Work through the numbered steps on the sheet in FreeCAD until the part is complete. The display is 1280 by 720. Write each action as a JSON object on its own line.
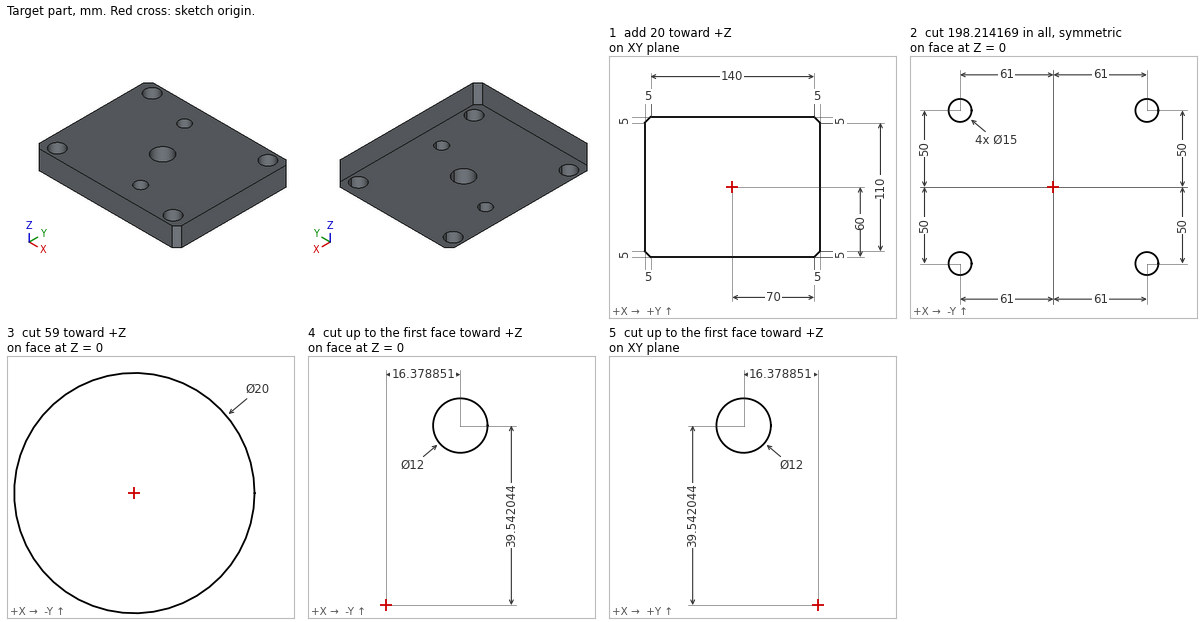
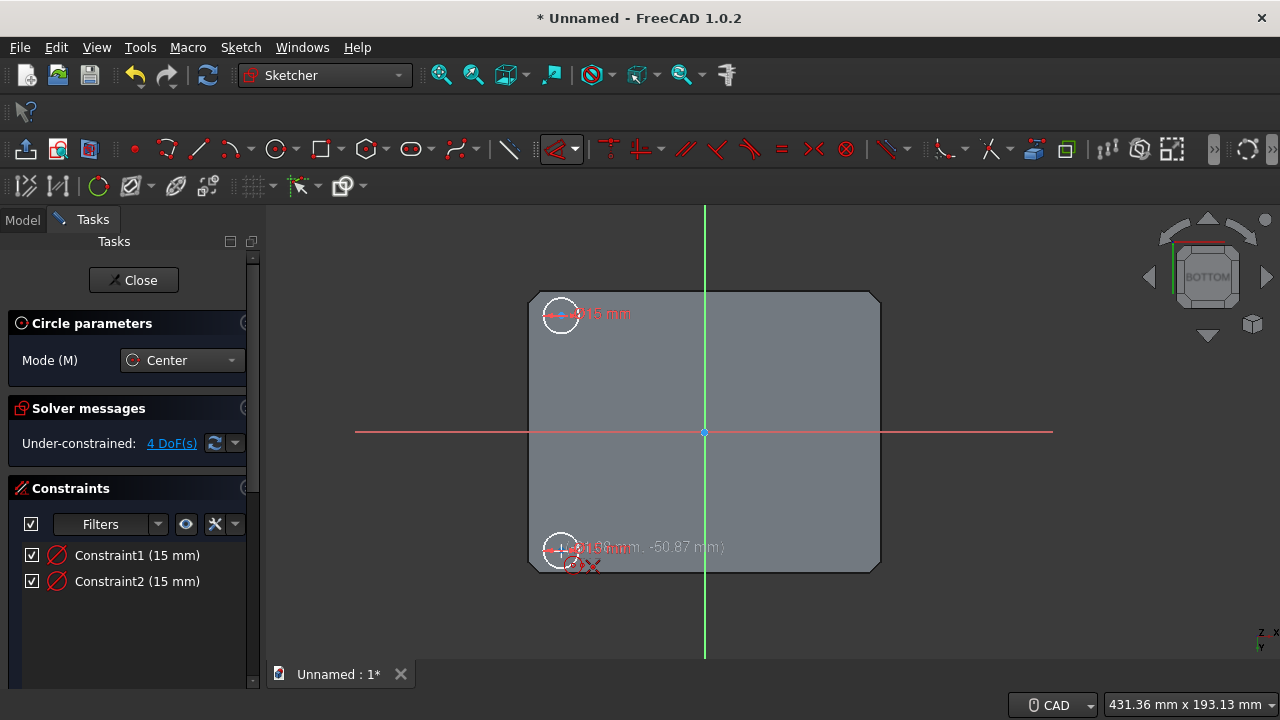
{"action": "scroll", "coordinate": [848, 315], "scroll_direction": "up", "scroll_amount": 2}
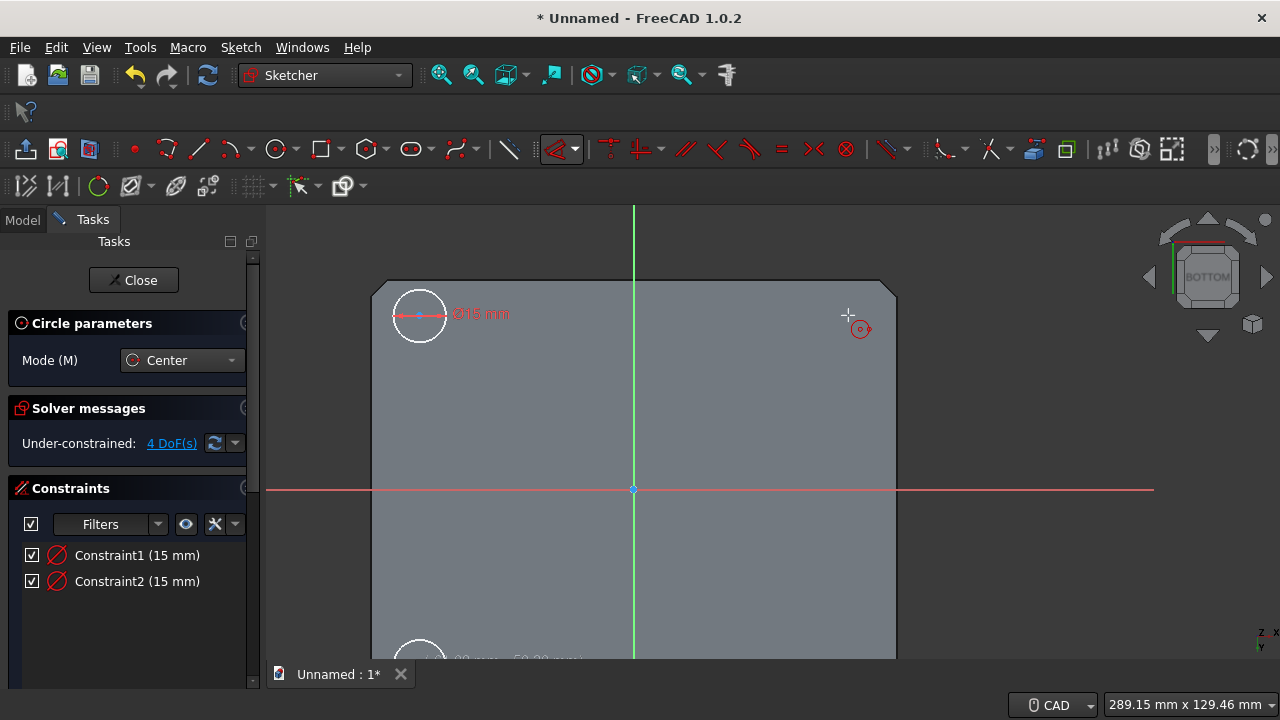
{"action": "left_click", "coordinate": [848, 315]}
{"action": "mouse_move", "coordinate": [866, 296]}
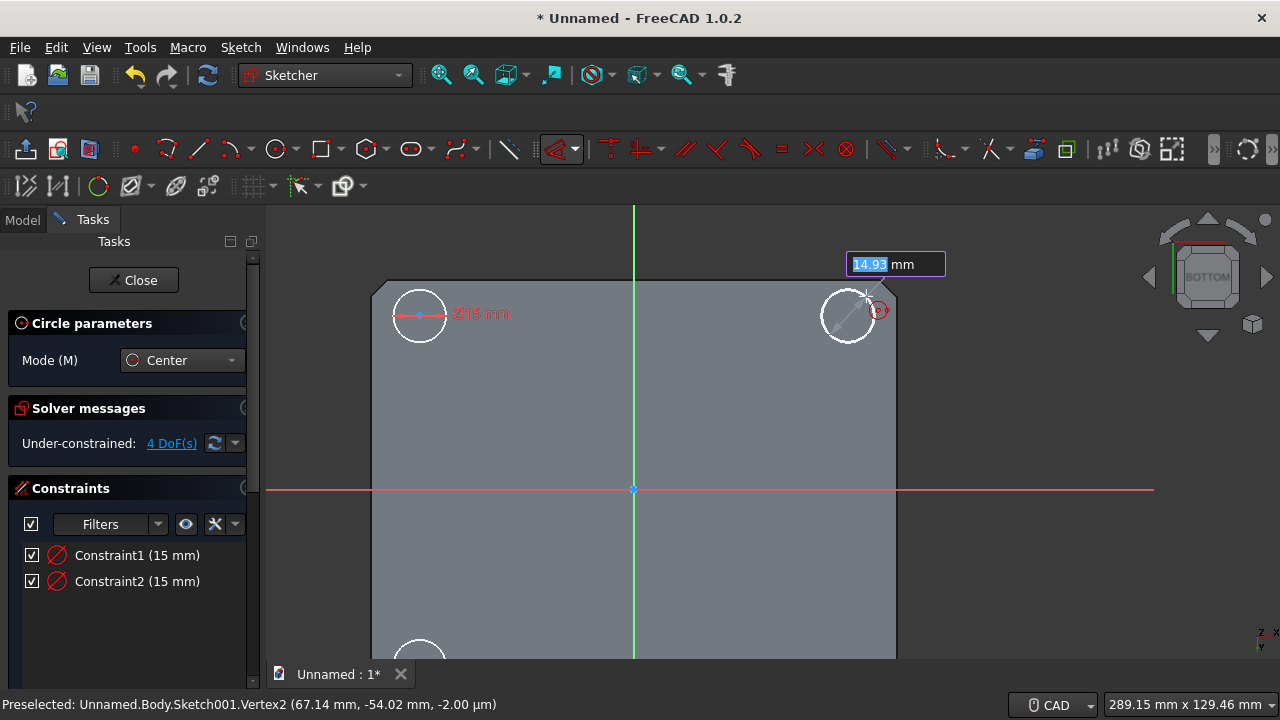
{"action": "type", "text": "15"}
{"action": "key", "text": "Return"}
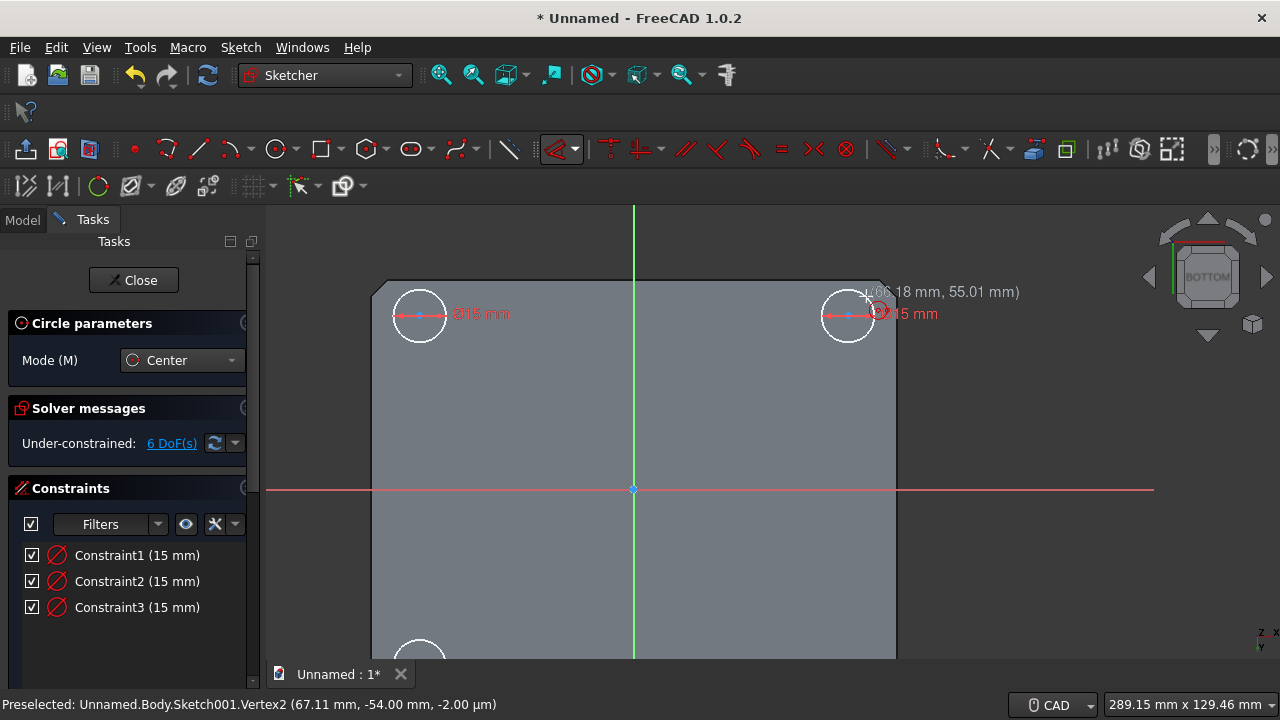
{"action": "scroll", "coordinate": [848, 314], "scroll_direction": "down", "scroll_amount": 2}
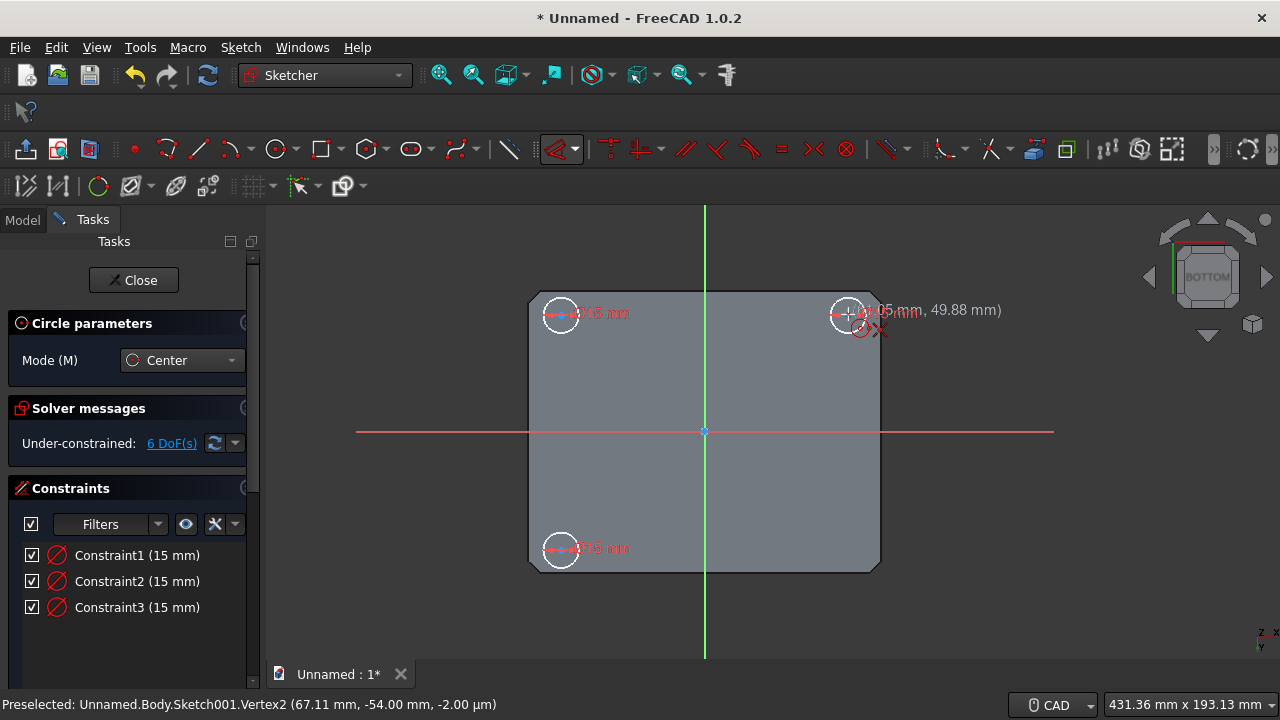
{"action": "scroll", "coordinate": [848, 550], "scroll_direction": "up", "scroll_amount": 2}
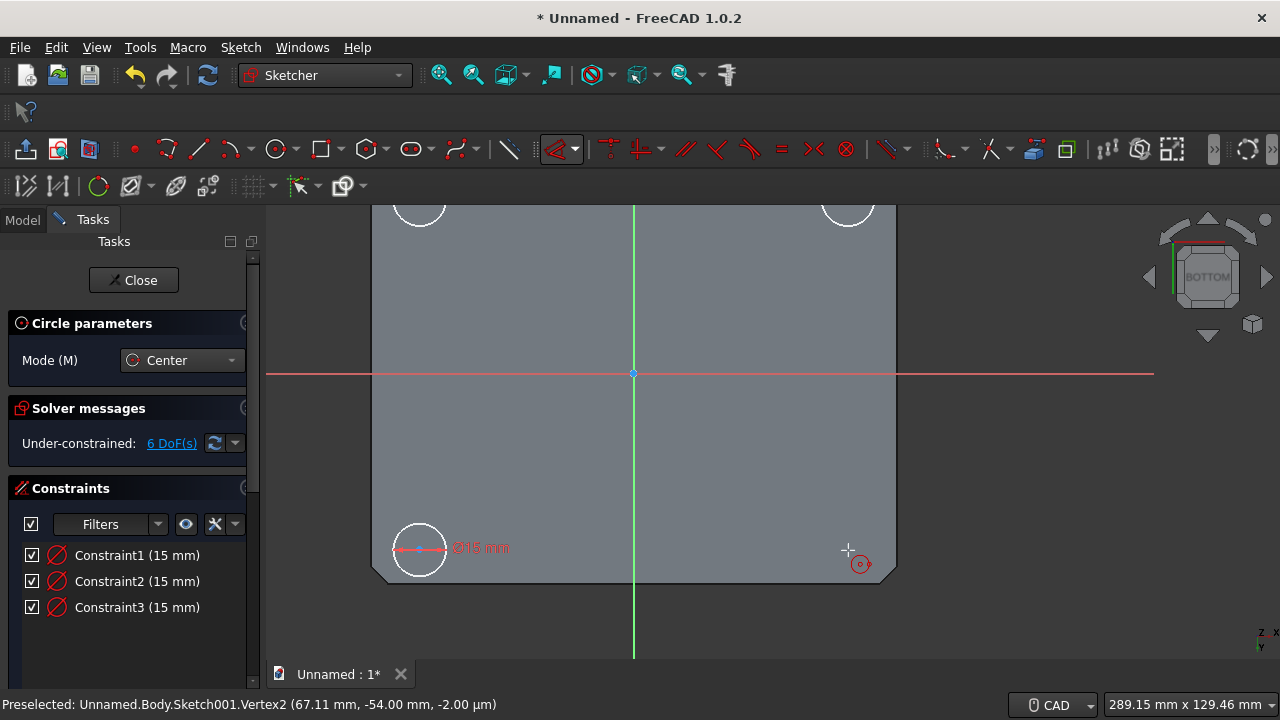
{"action": "left_click", "coordinate": [848, 549]}
{"action": "mouse_move", "coordinate": [866, 530]}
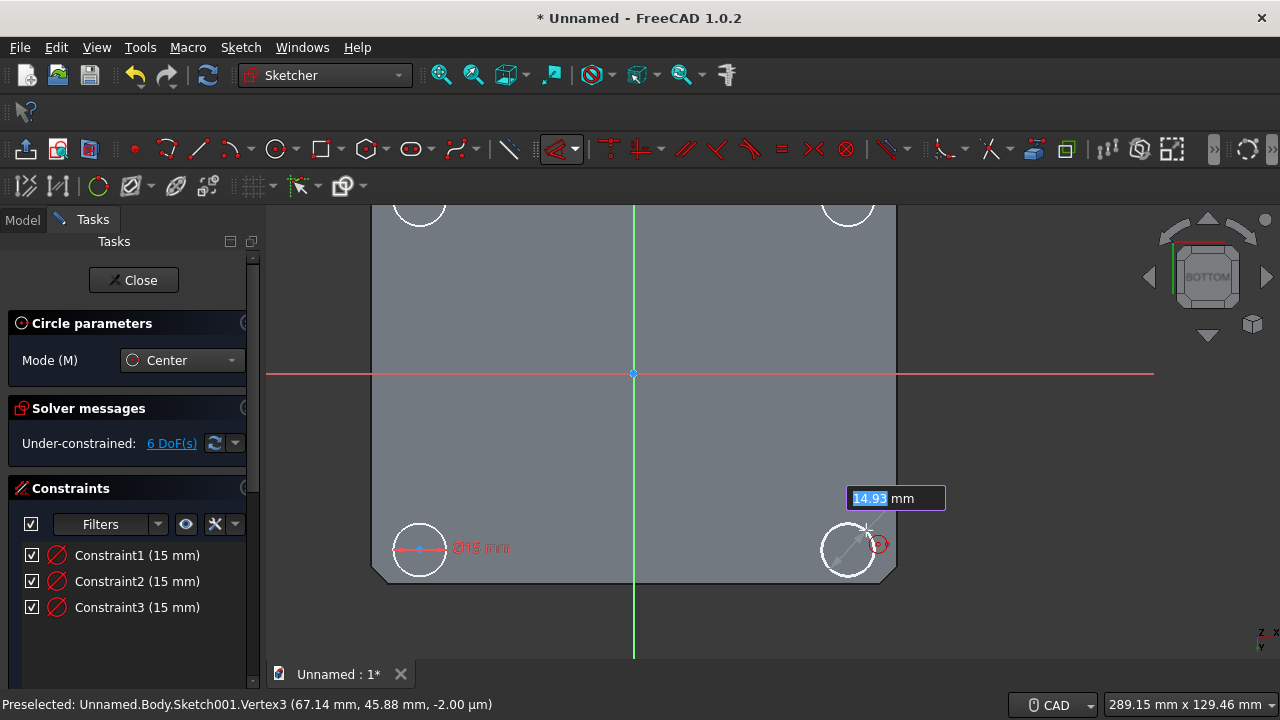
{"action": "type", "text": "15"}
{"action": "key", "text": "Return"}
{"action": "key", "text": "Escape"}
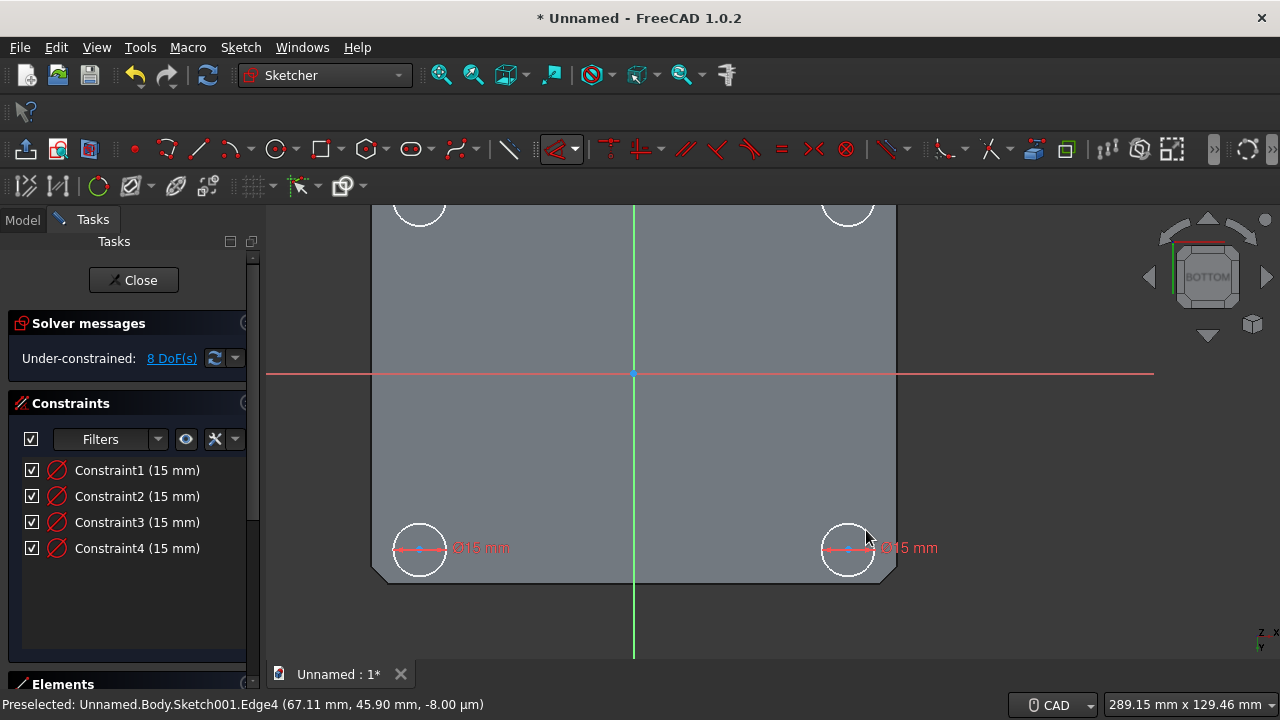
{"action": "scroll", "coordinate": [848, 551], "scroll_direction": "down", "scroll_amount": 2}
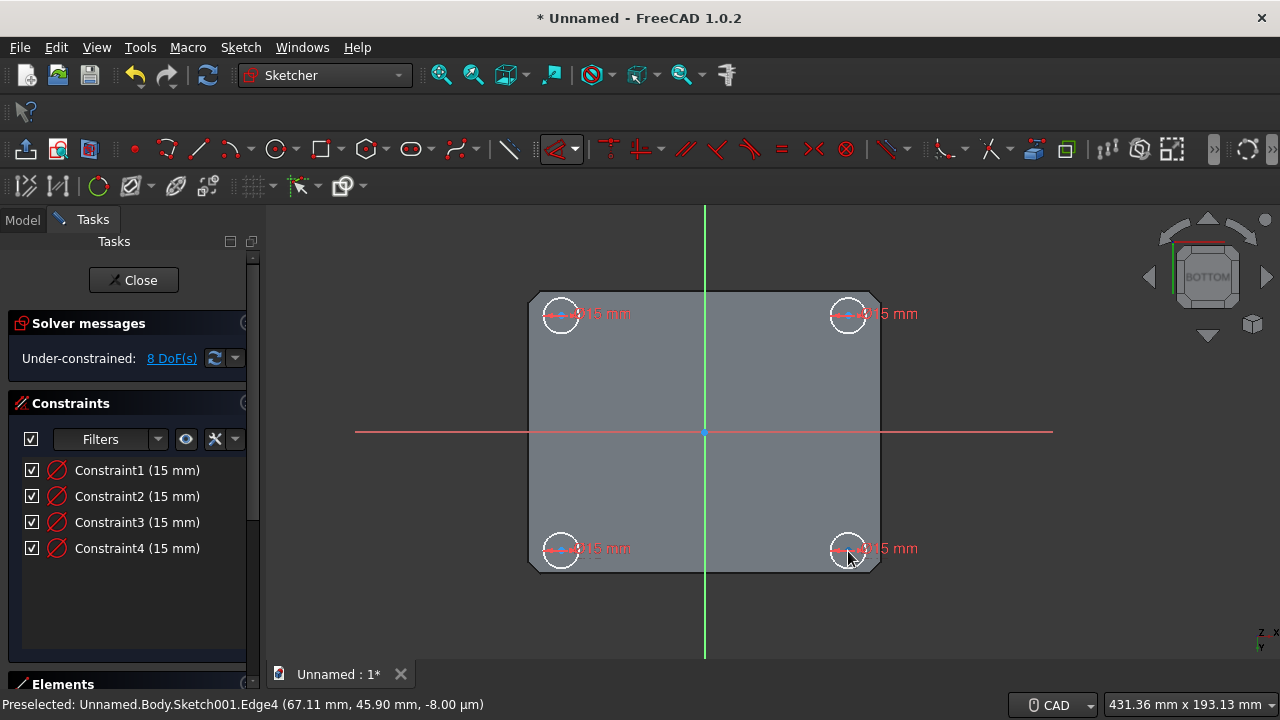
{"action": "left_click", "coordinate": [561, 316]}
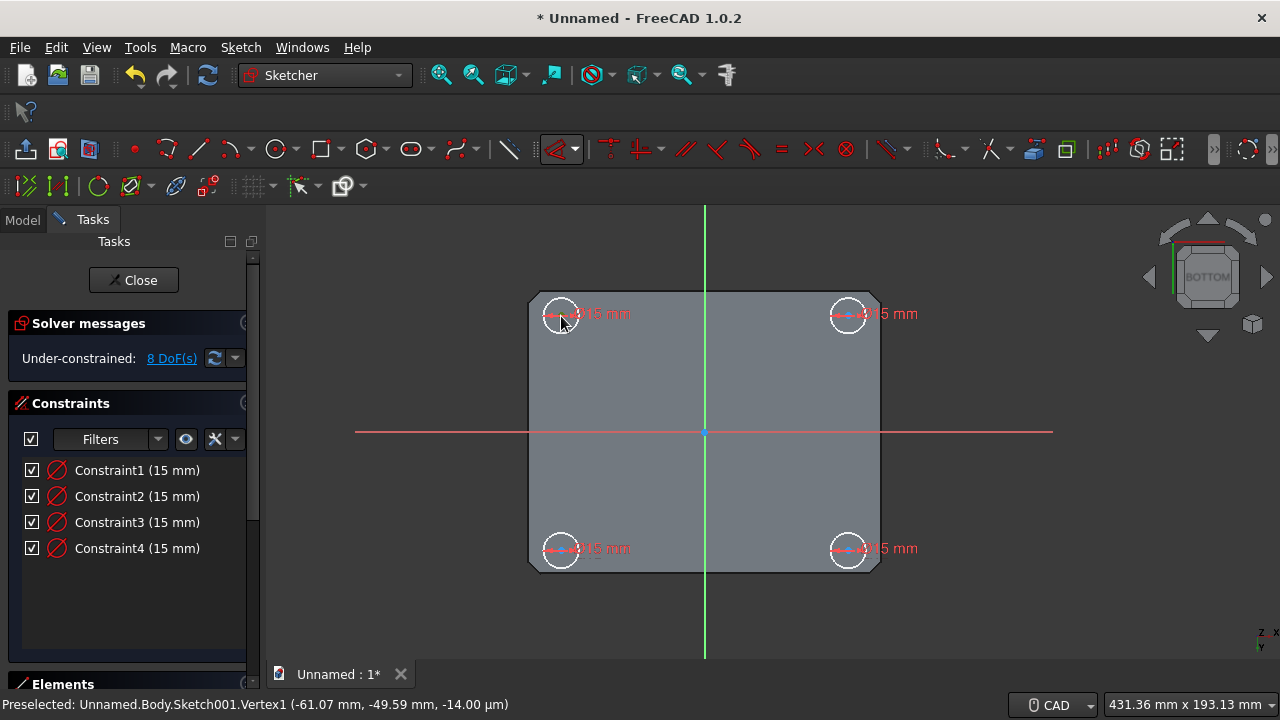
{"action": "left_click", "coordinate": [578, 150]}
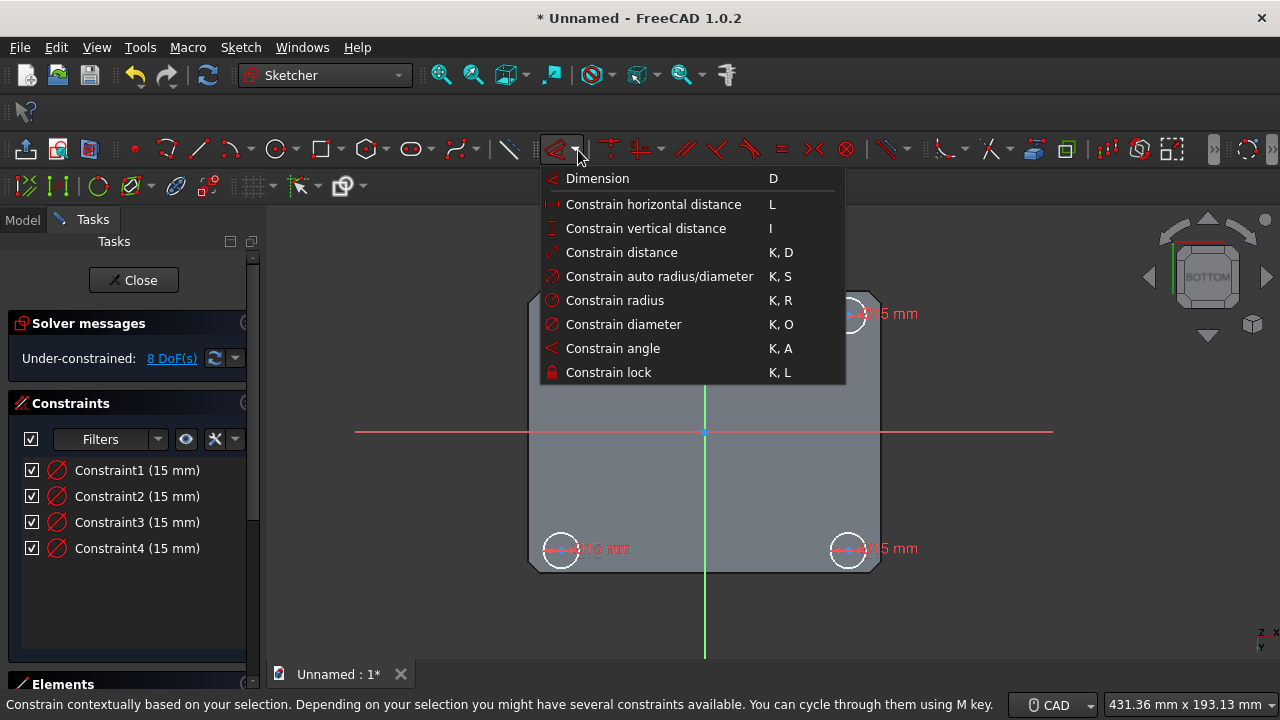
{"action": "left_click", "coordinate": [693, 204]}